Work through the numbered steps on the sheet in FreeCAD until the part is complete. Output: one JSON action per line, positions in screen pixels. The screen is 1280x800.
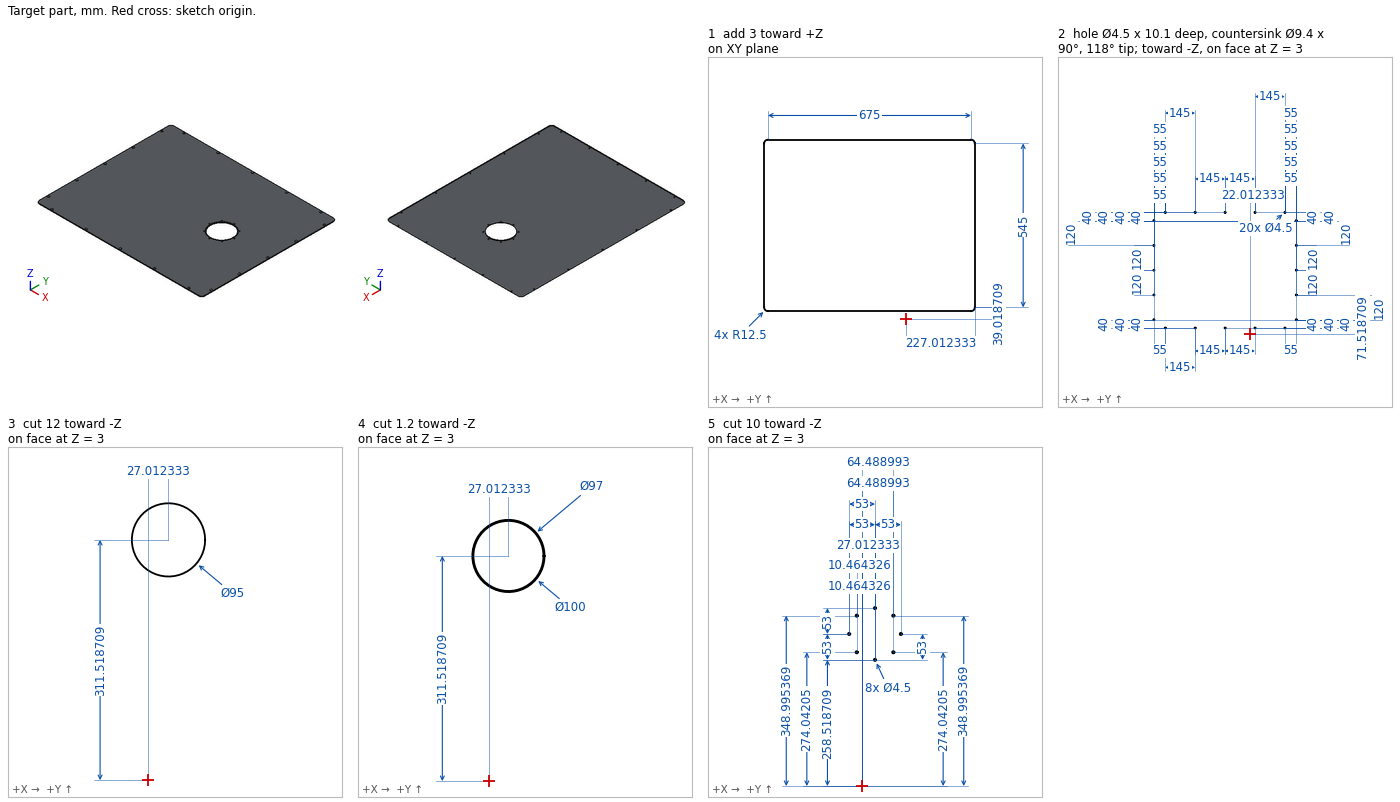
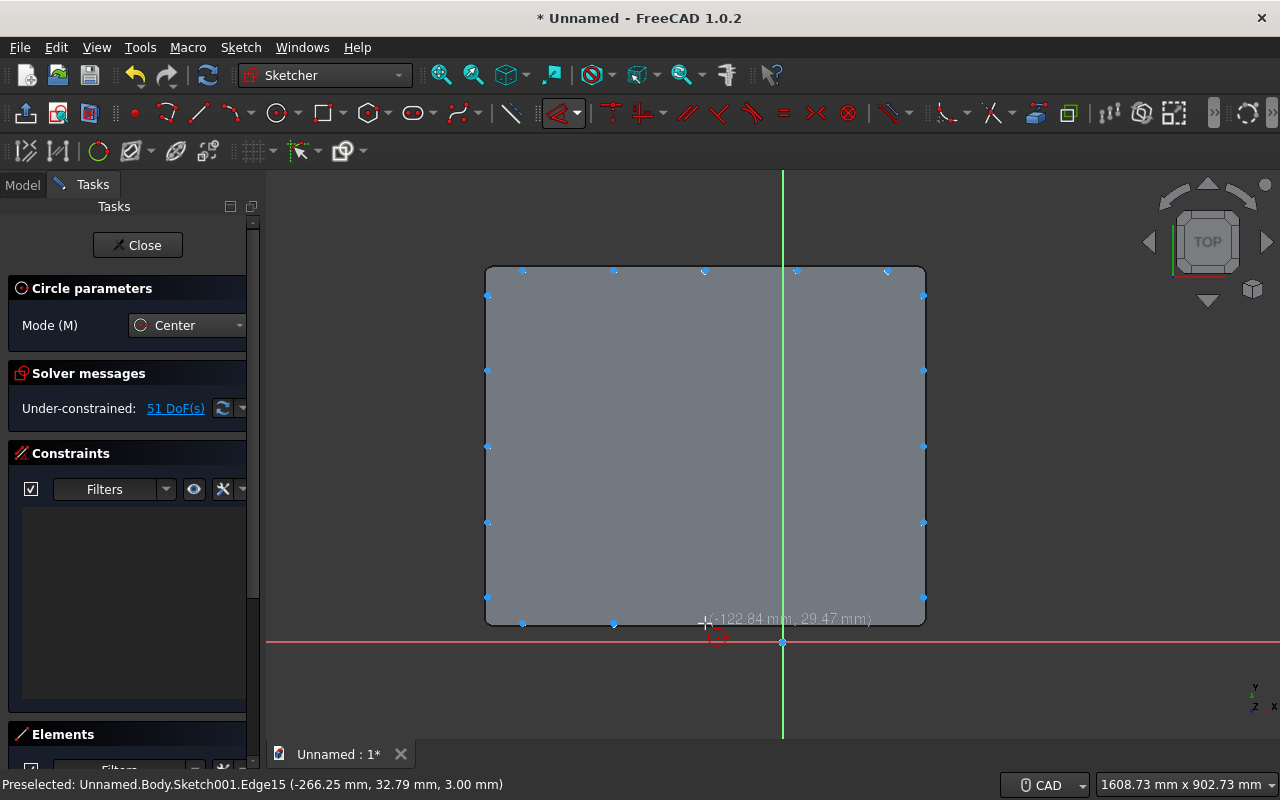
{"action": "left_click", "coordinate": [705, 623]}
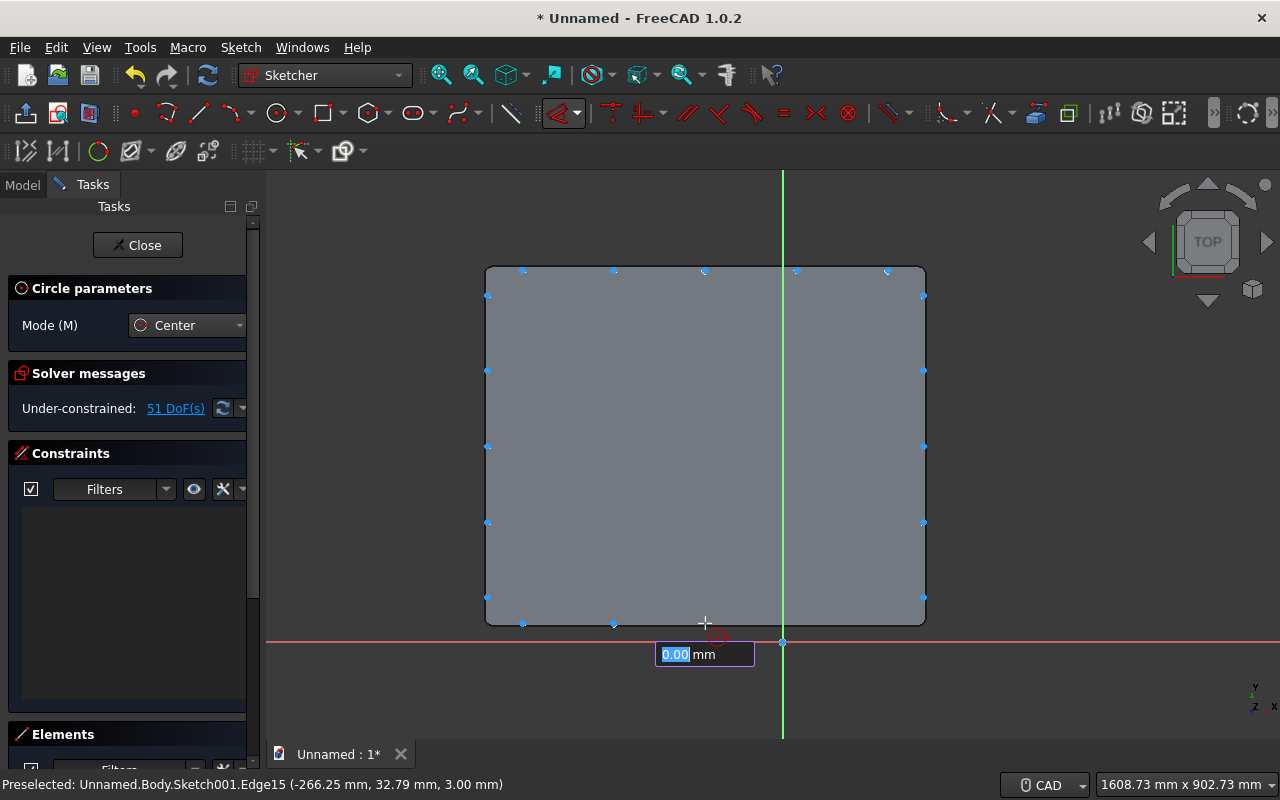
{"action": "scroll", "coordinate": [706, 622], "scroll_direction": "up", "scroll_amount": 13}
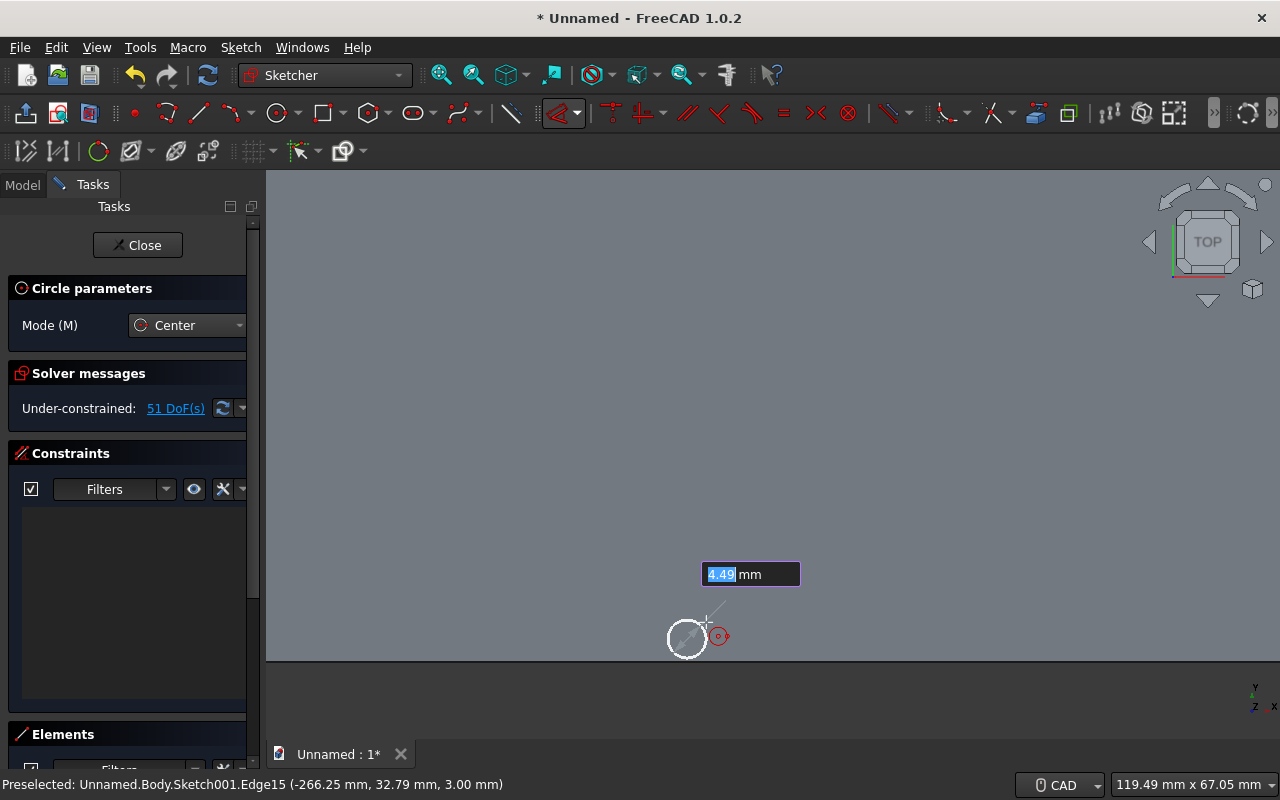
{"action": "left_click", "coordinate": [705, 606]}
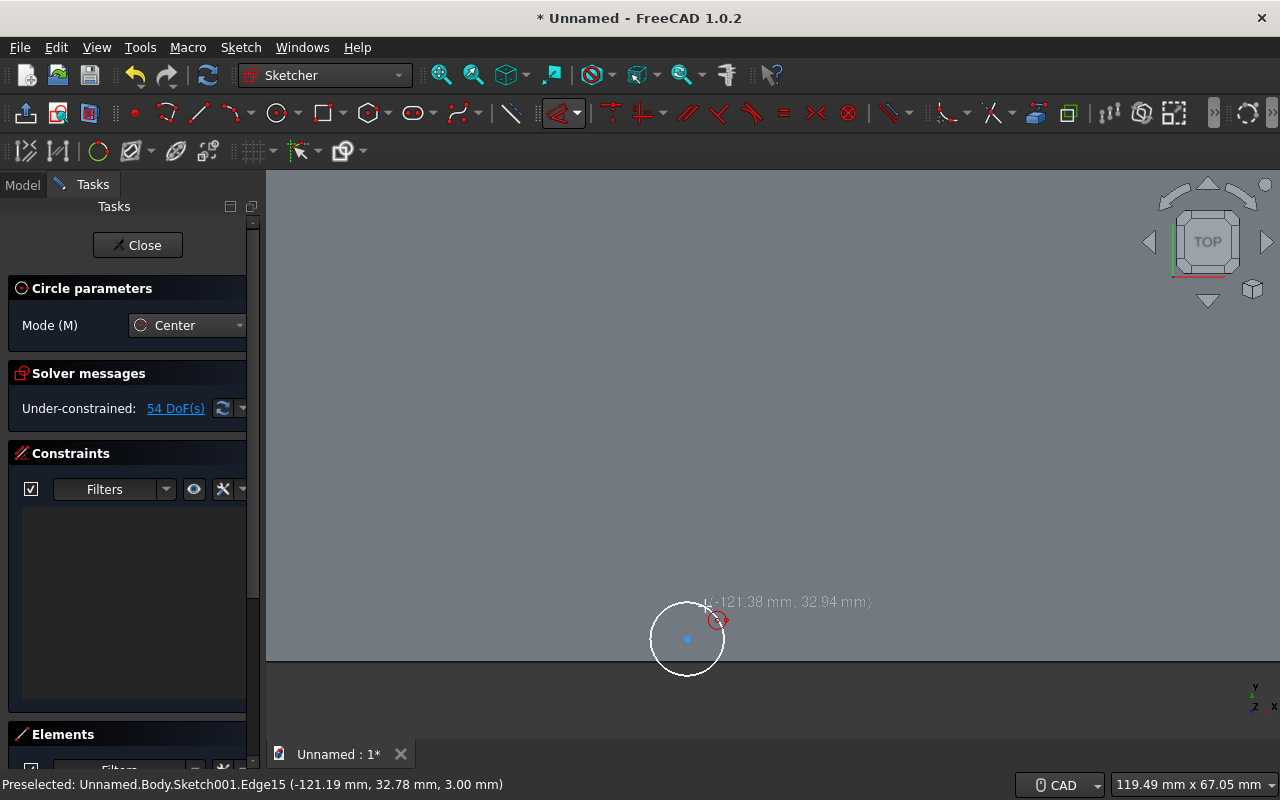
{"action": "scroll", "coordinate": [706, 622], "scroll_direction": "down", "scroll_amount": 13}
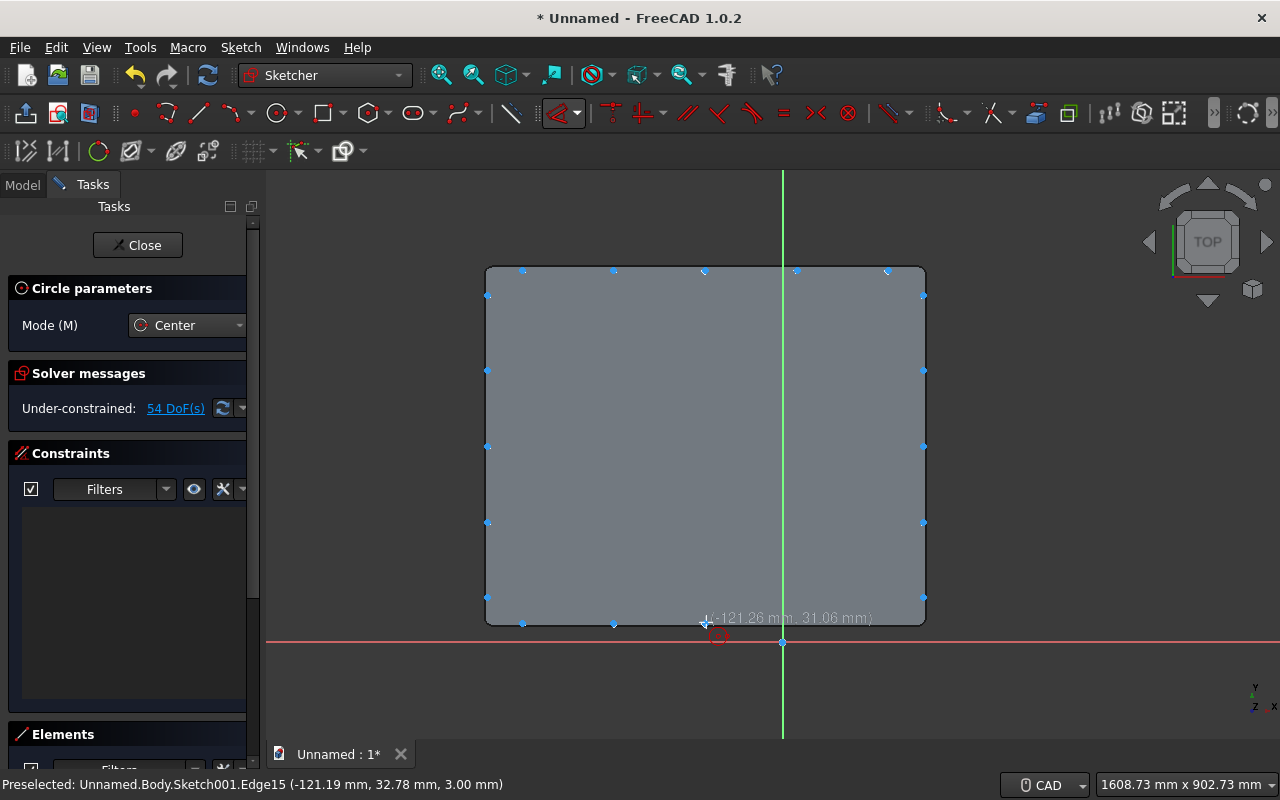
{"action": "scroll", "coordinate": [797, 623], "scroll_direction": "up", "scroll_amount": 14}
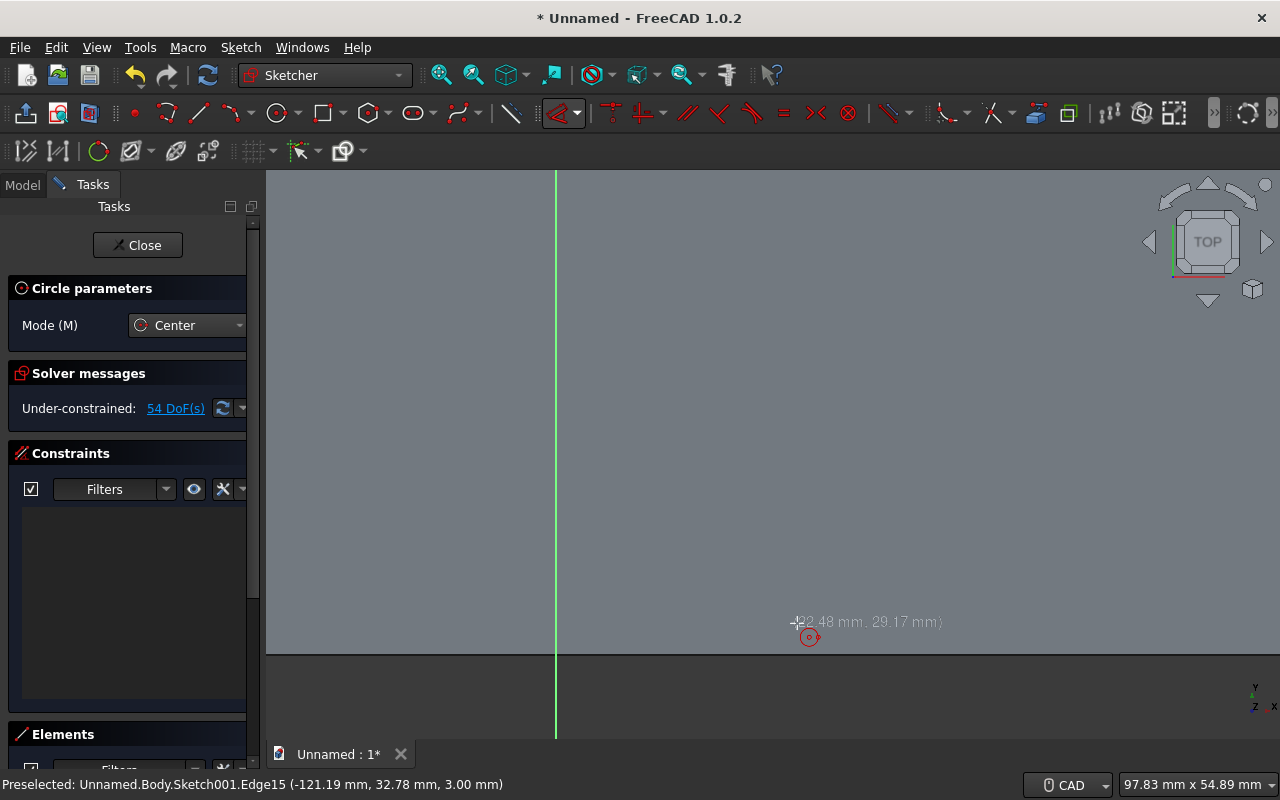
{"action": "scroll", "coordinate": [797, 623], "scroll_direction": "down", "scroll_amount": 14}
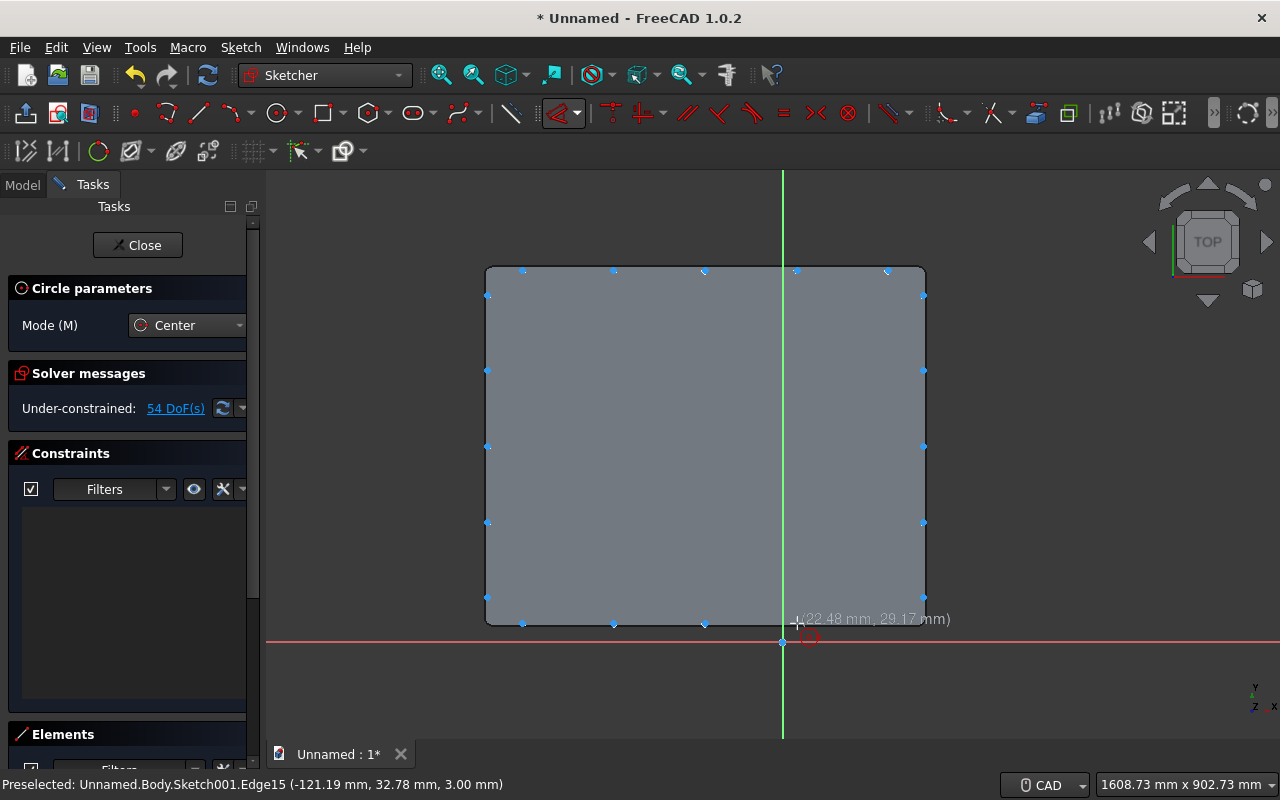
{"action": "left_click", "coordinate": [797, 623]}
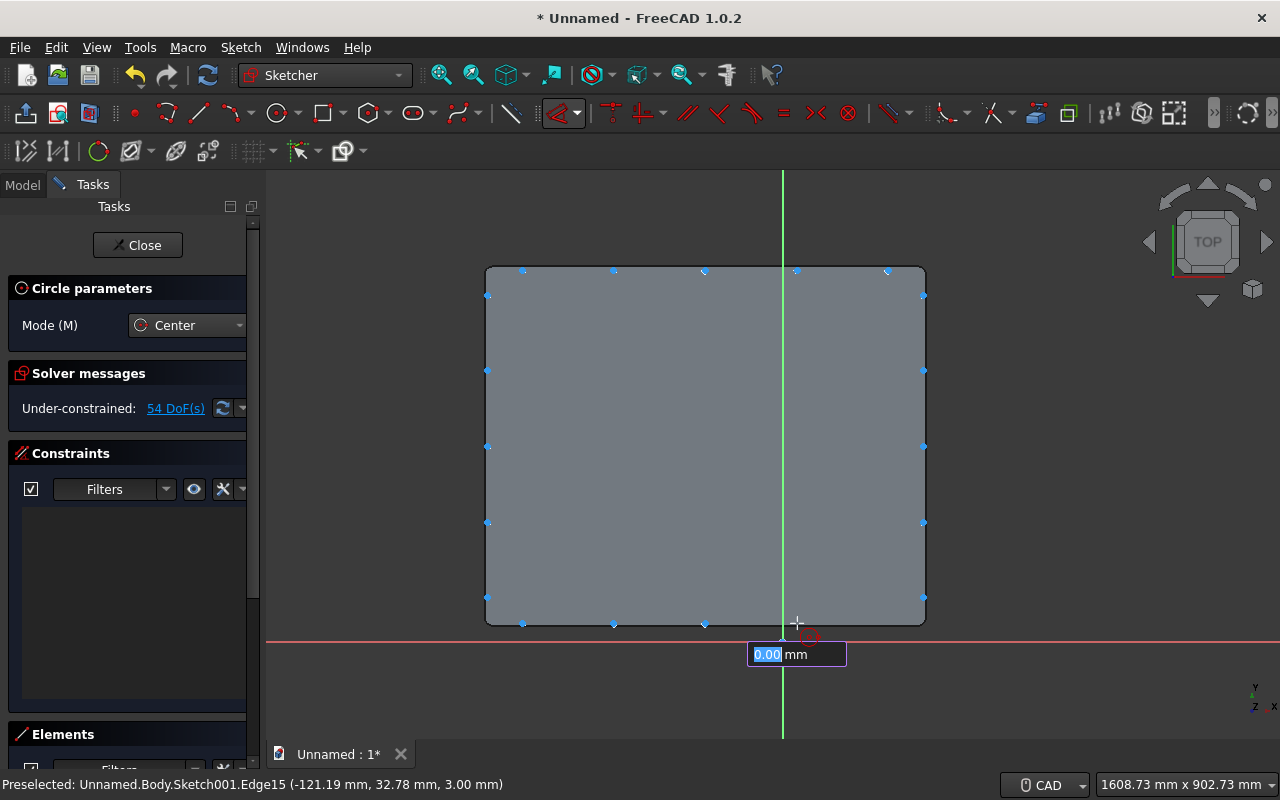
{"action": "scroll", "coordinate": [798, 622], "scroll_direction": "up", "scroll_amount": 13}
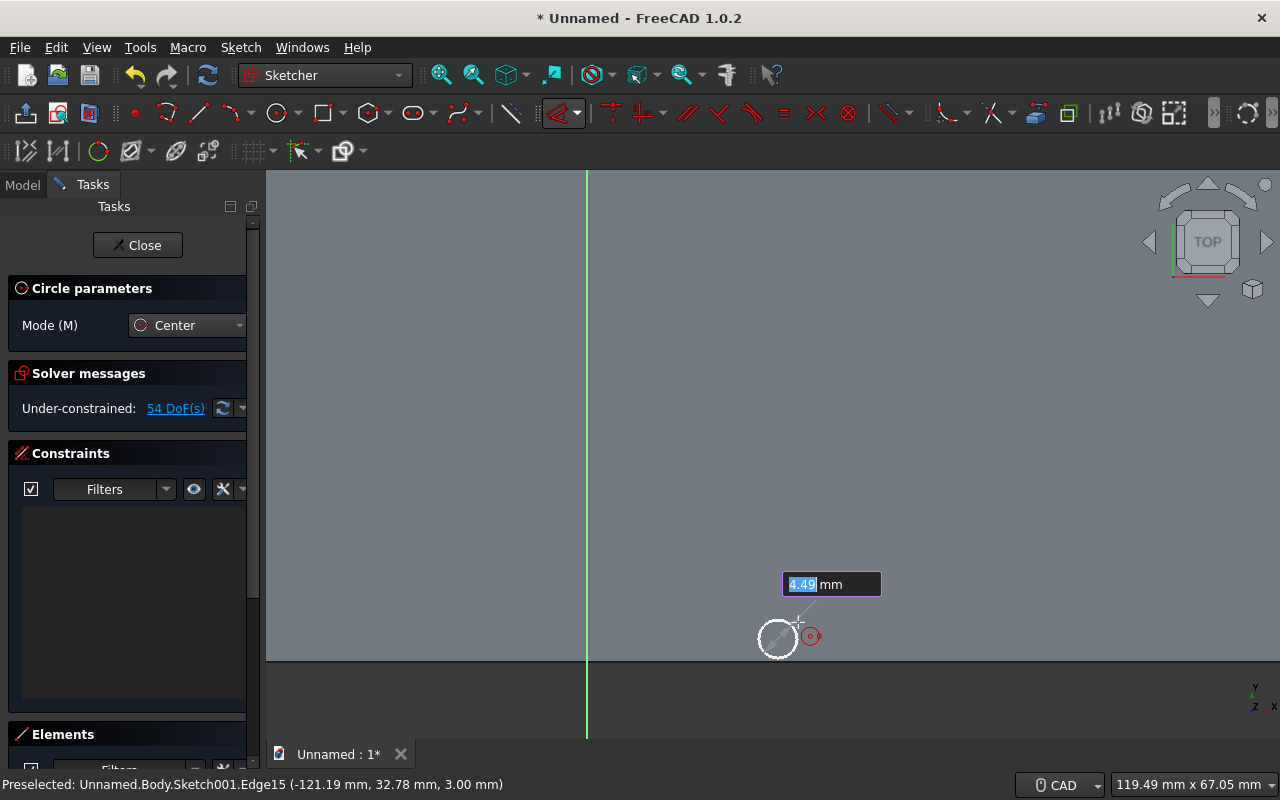
{"action": "left_click", "coordinate": [788, 606]}